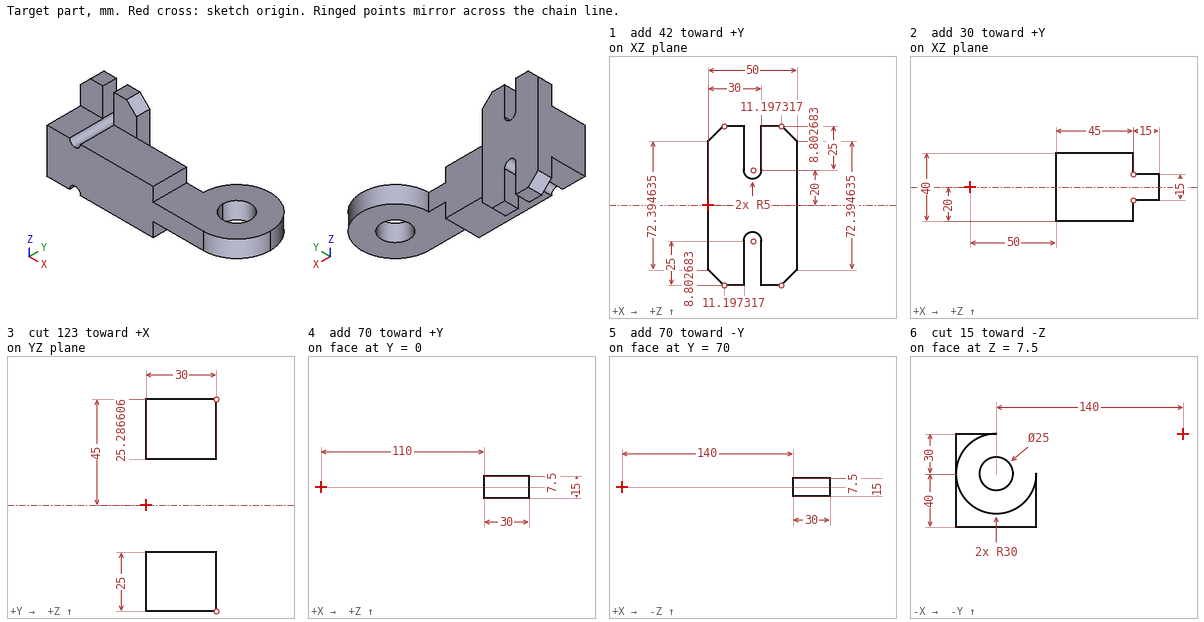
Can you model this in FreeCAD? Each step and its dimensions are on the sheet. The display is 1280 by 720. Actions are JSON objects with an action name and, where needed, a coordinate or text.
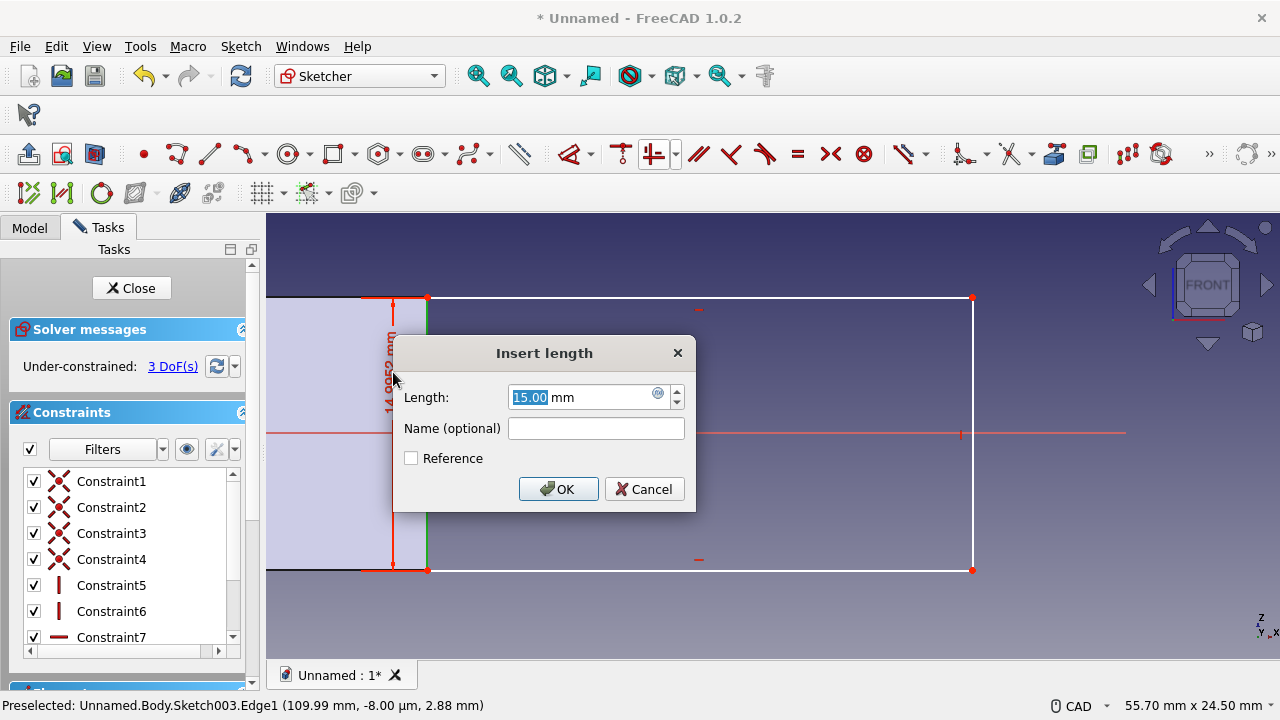
{"action": "type", "text": "15"}
{"action": "key", "text": "Return"}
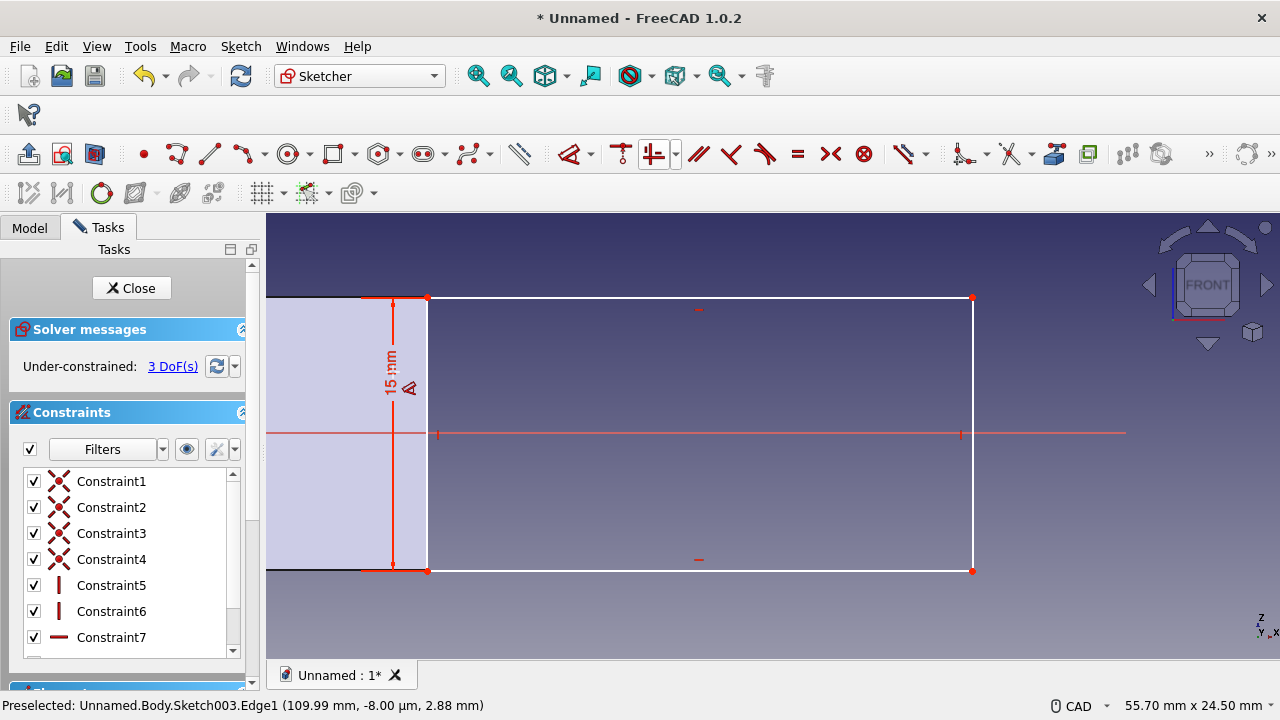
{"action": "left_click", "coordinate": [591, 571]}
{"action": "left_click", "coordinate": [700, 605]}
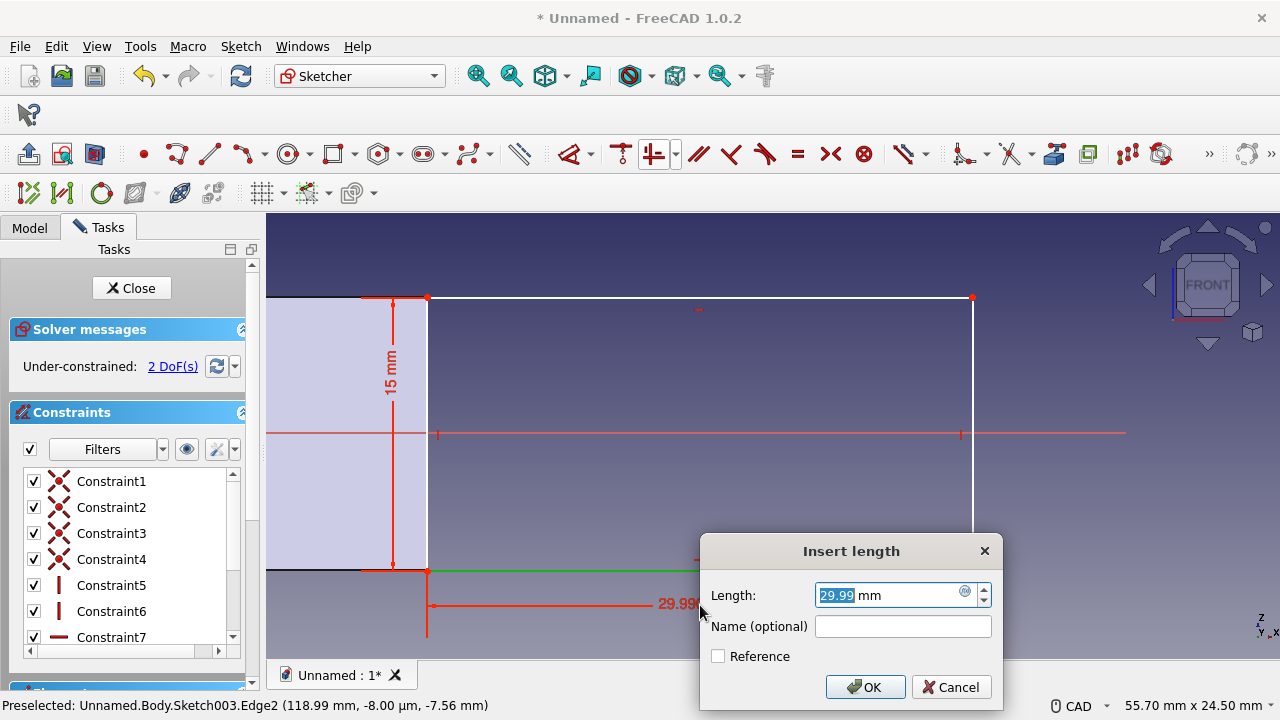
{"action": "type", "text": "30"}
{"action": "key", "text": "Return"}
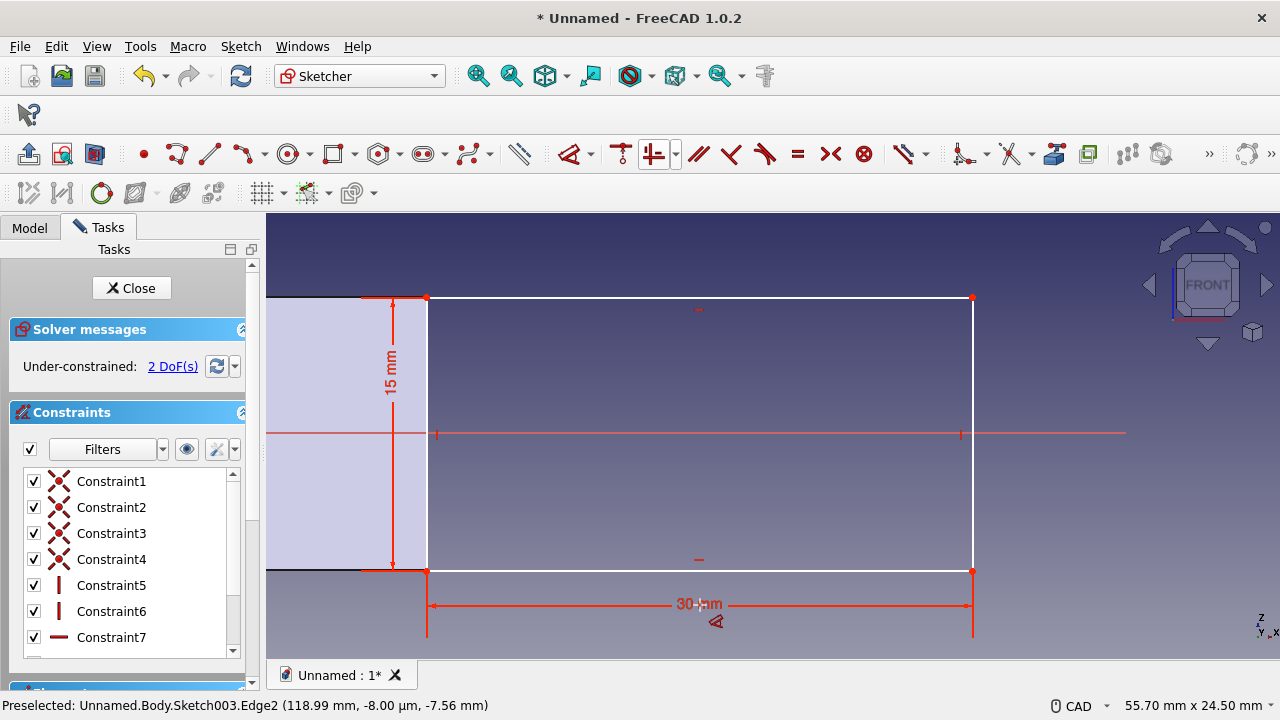
{"action": "left_click", "coordinate": [427, 298]}
{"action": "left_click", "coordinate": [360, 264]}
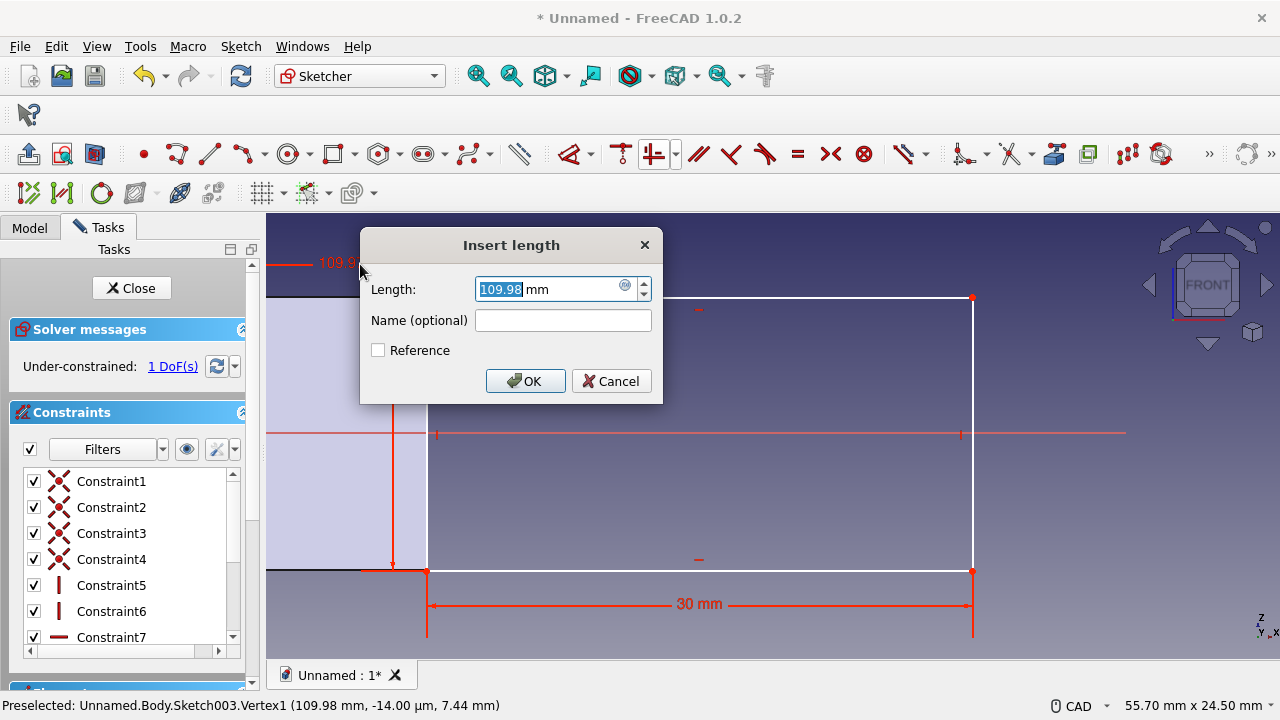
{"action": "type", "text": "110"}
{"action": "key", "text": "Return"}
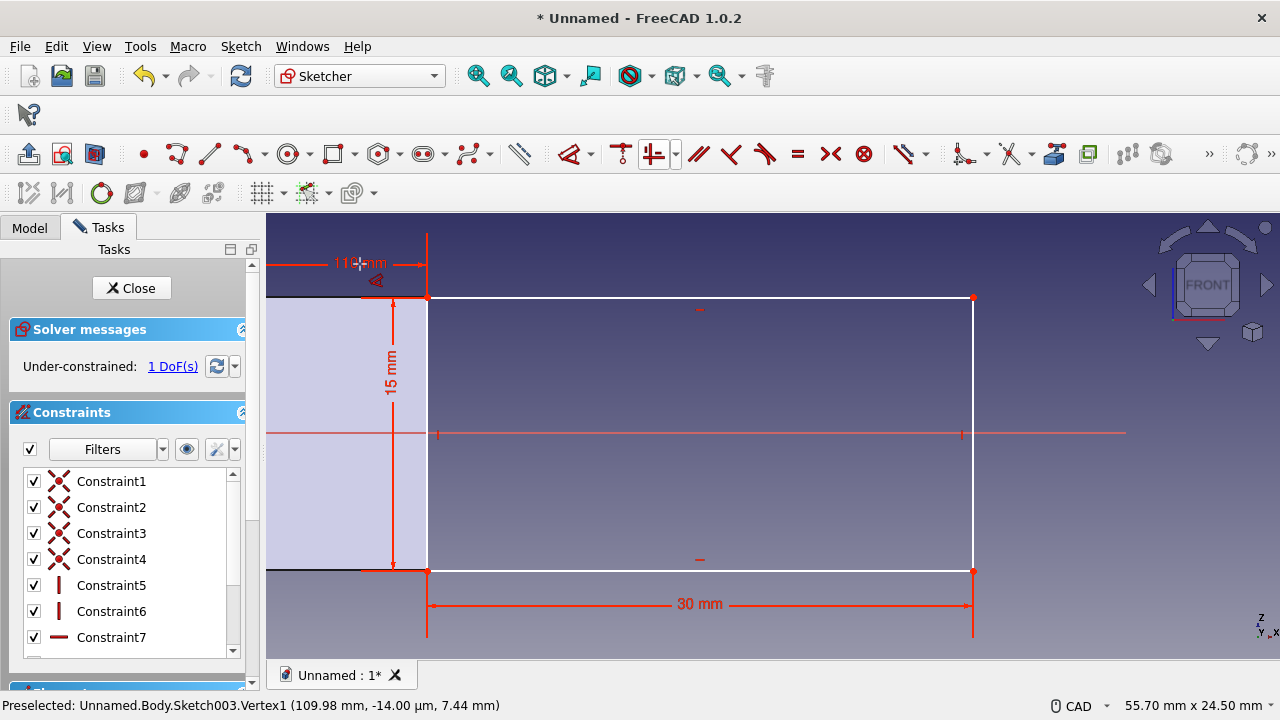
{"action": "left_click", "coordinate": [427, 298]}
{"action": "left_click", "coordinate": [461, 335]}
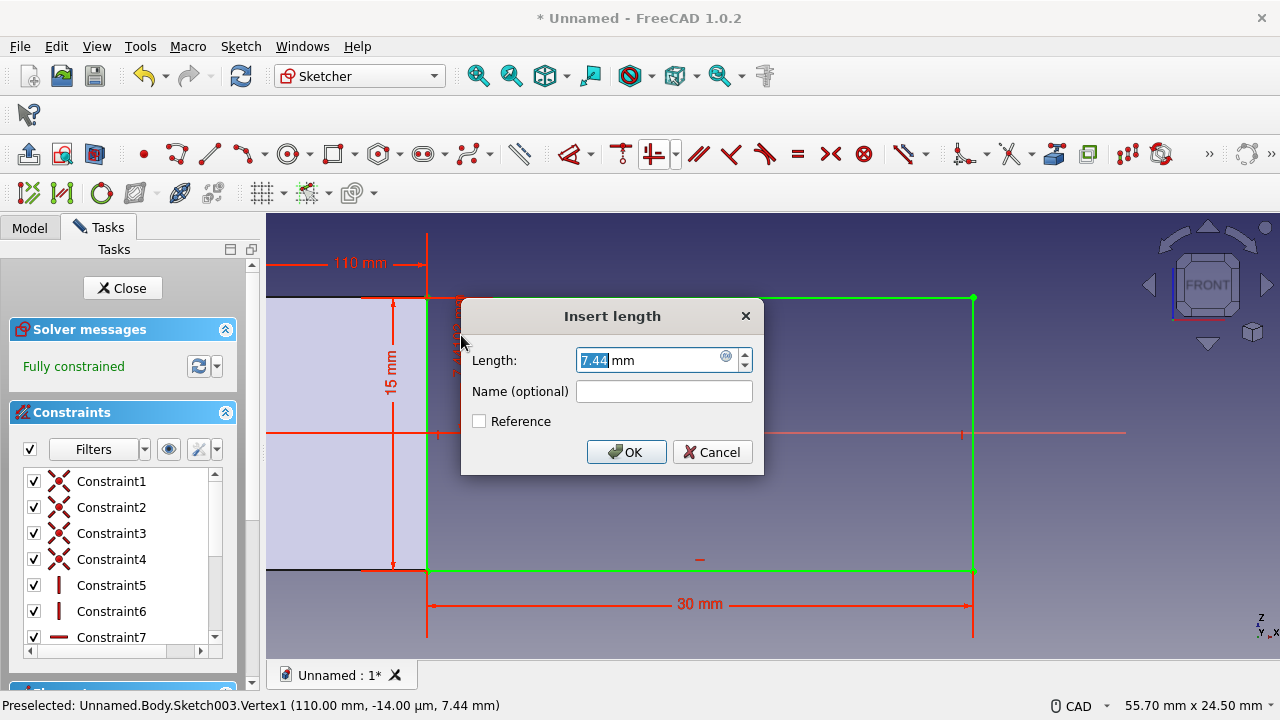
{"action": "type", "text": "7.5"}
{"action": "key", "text": "Return"}
{"action": "key", "text": "Escape"}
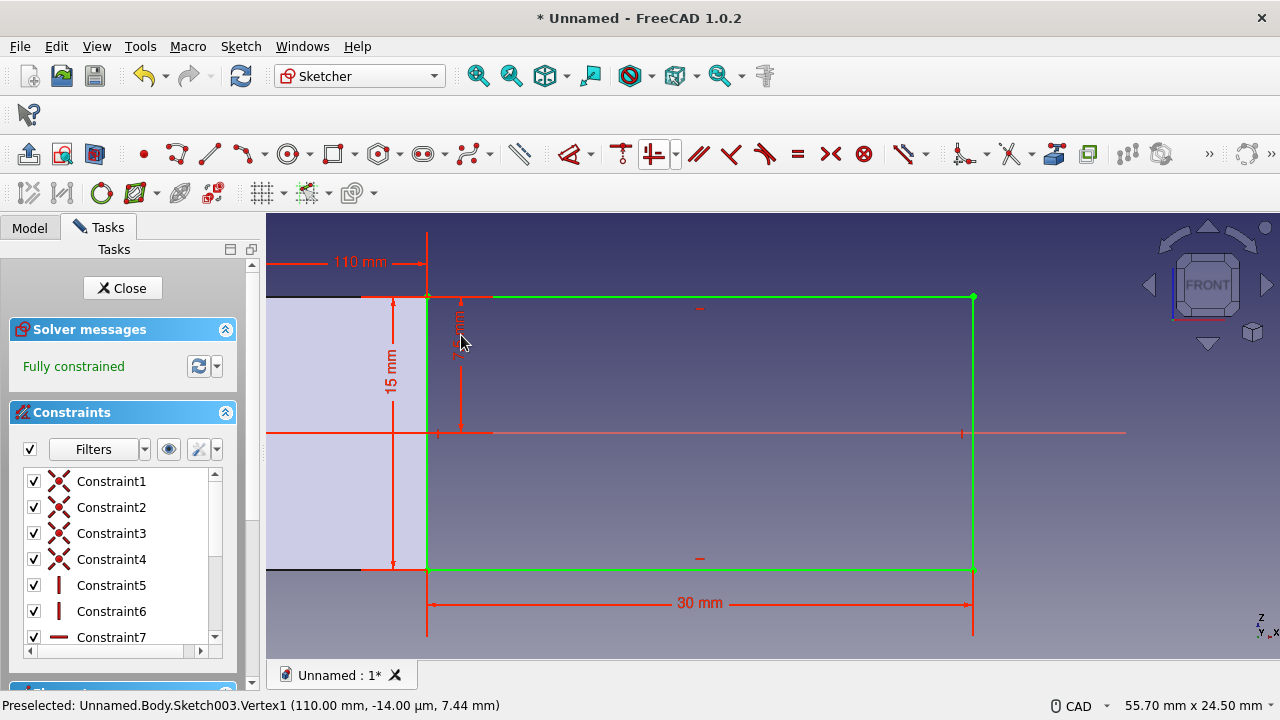
{"action": "left_click", "coordinate": [123, 288]}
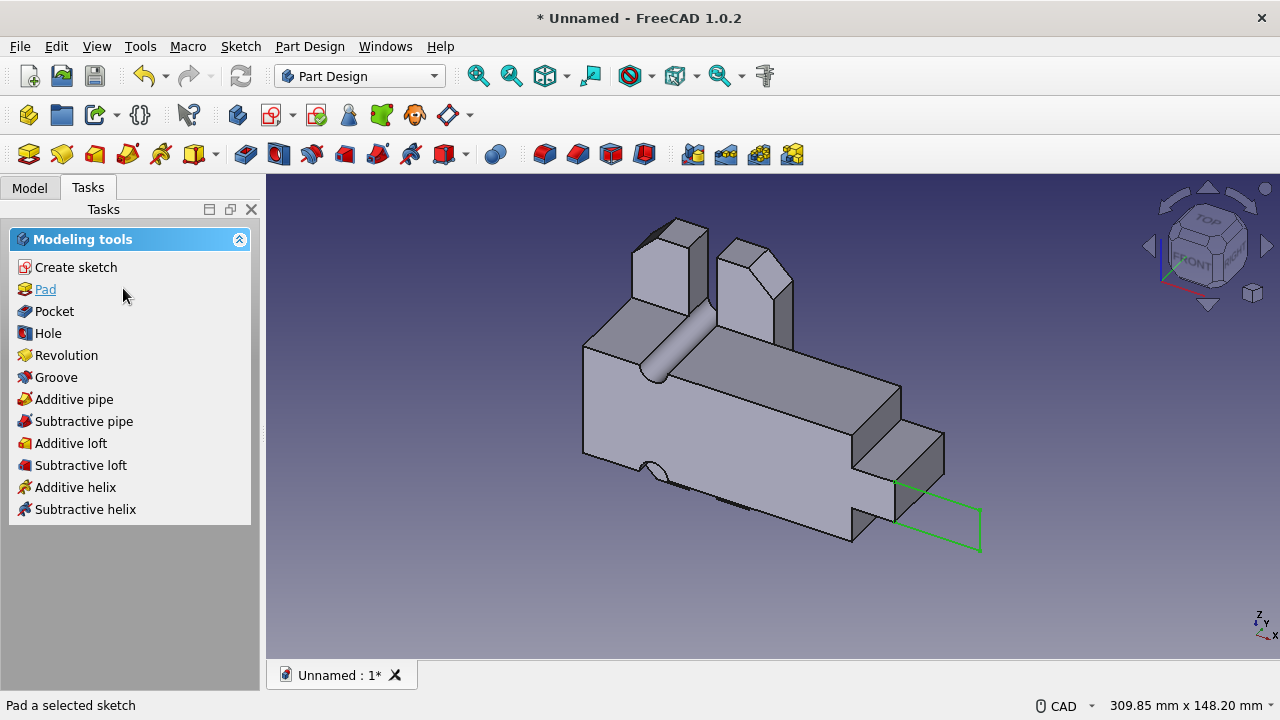
{"action": "left_click", "coordinate": [29, 154]}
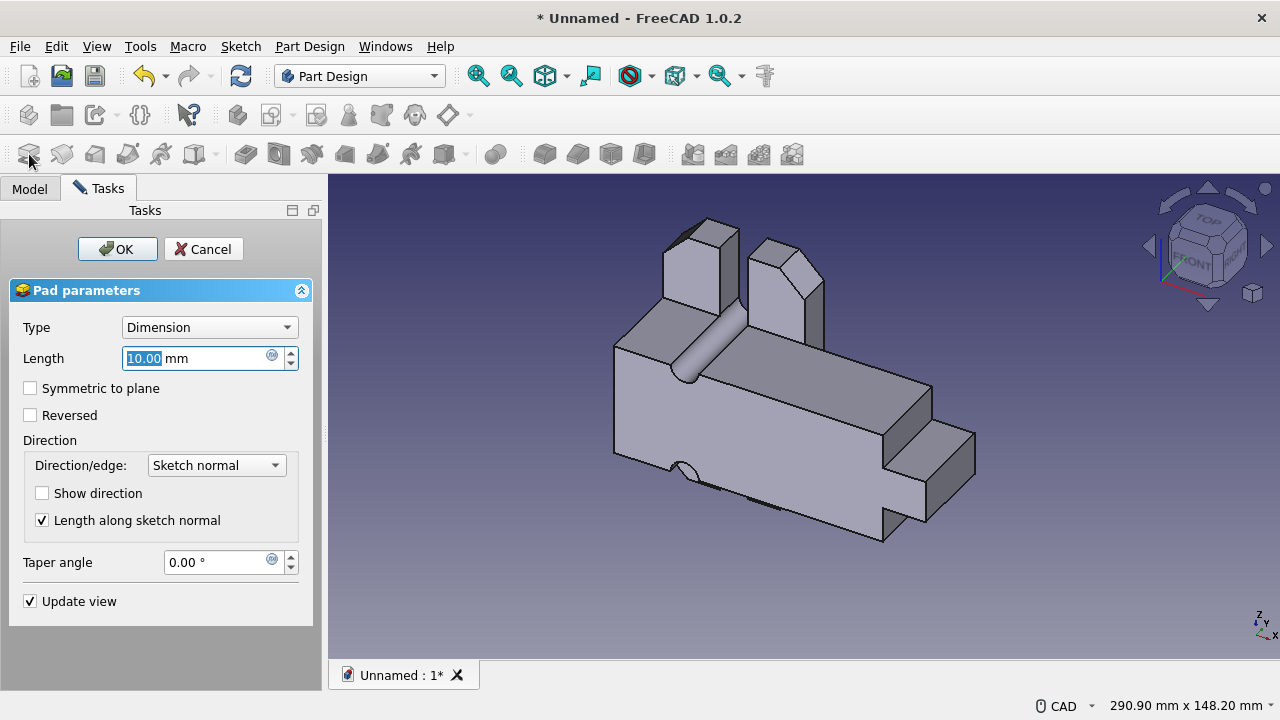
{"action": "type", "text": "70"}
{"action": "key", "text": "Tab"}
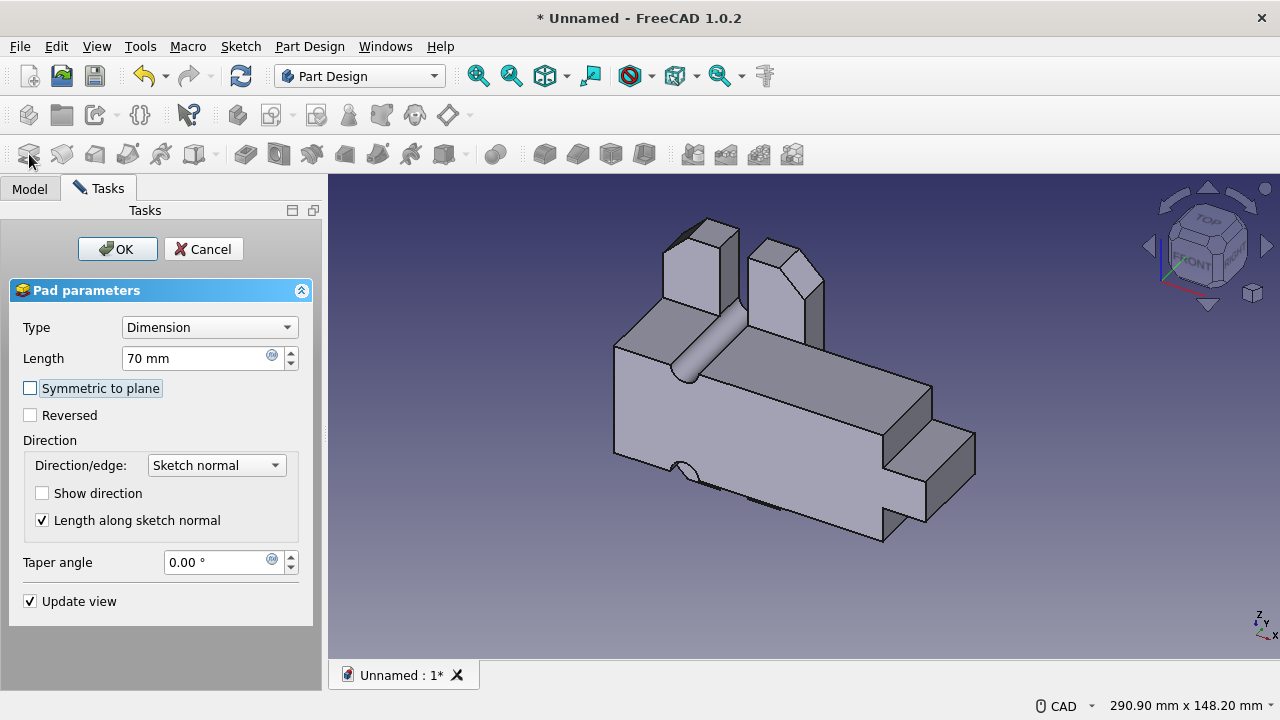
{"action": "left_click", "coordinate": [31, 415]}